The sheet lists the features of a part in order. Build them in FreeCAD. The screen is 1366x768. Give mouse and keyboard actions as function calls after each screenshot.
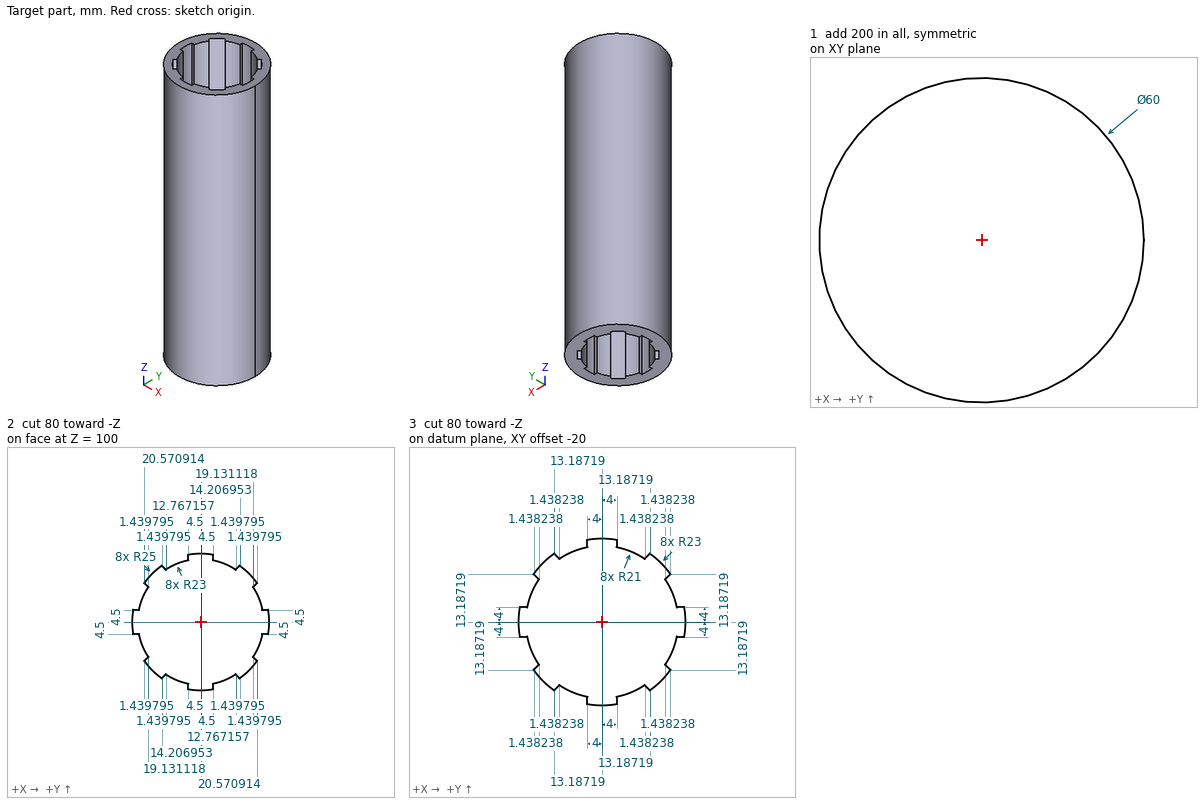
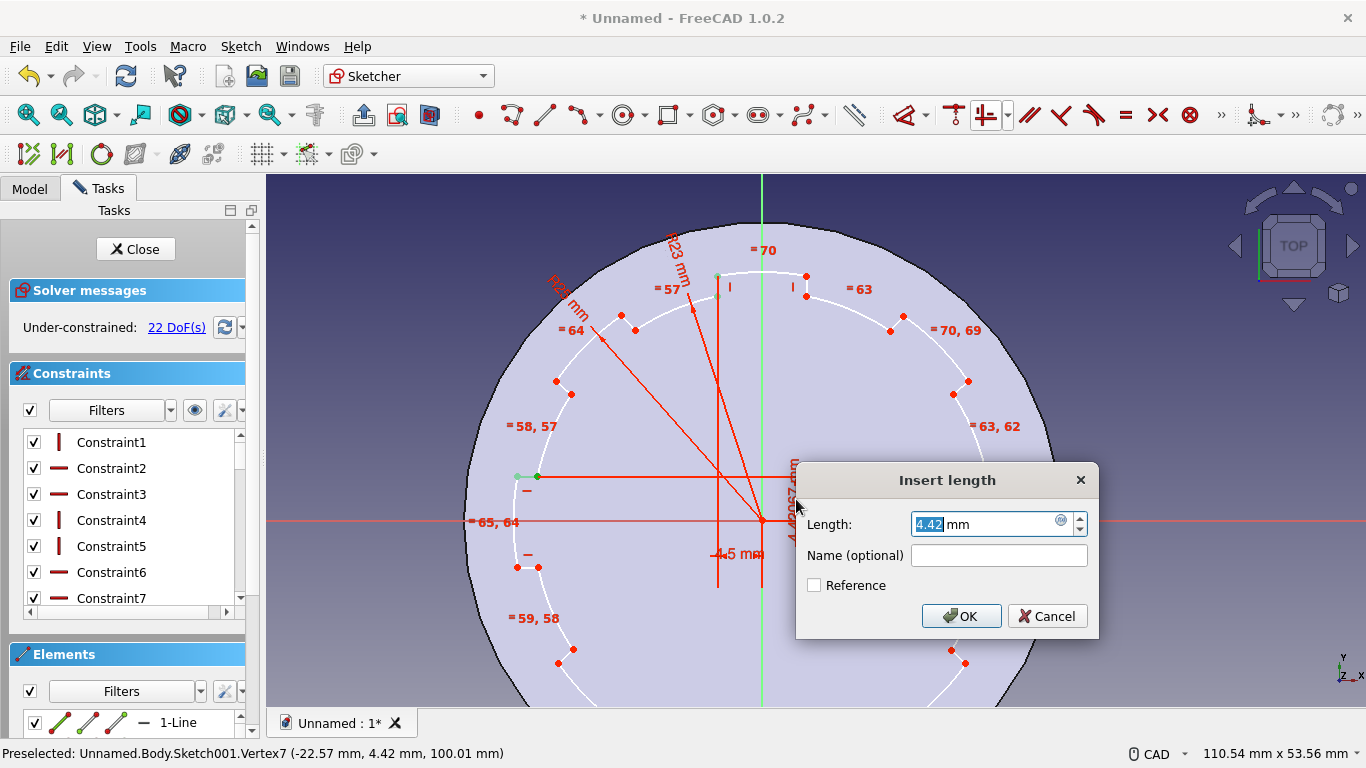
text(4.5)
key(Return)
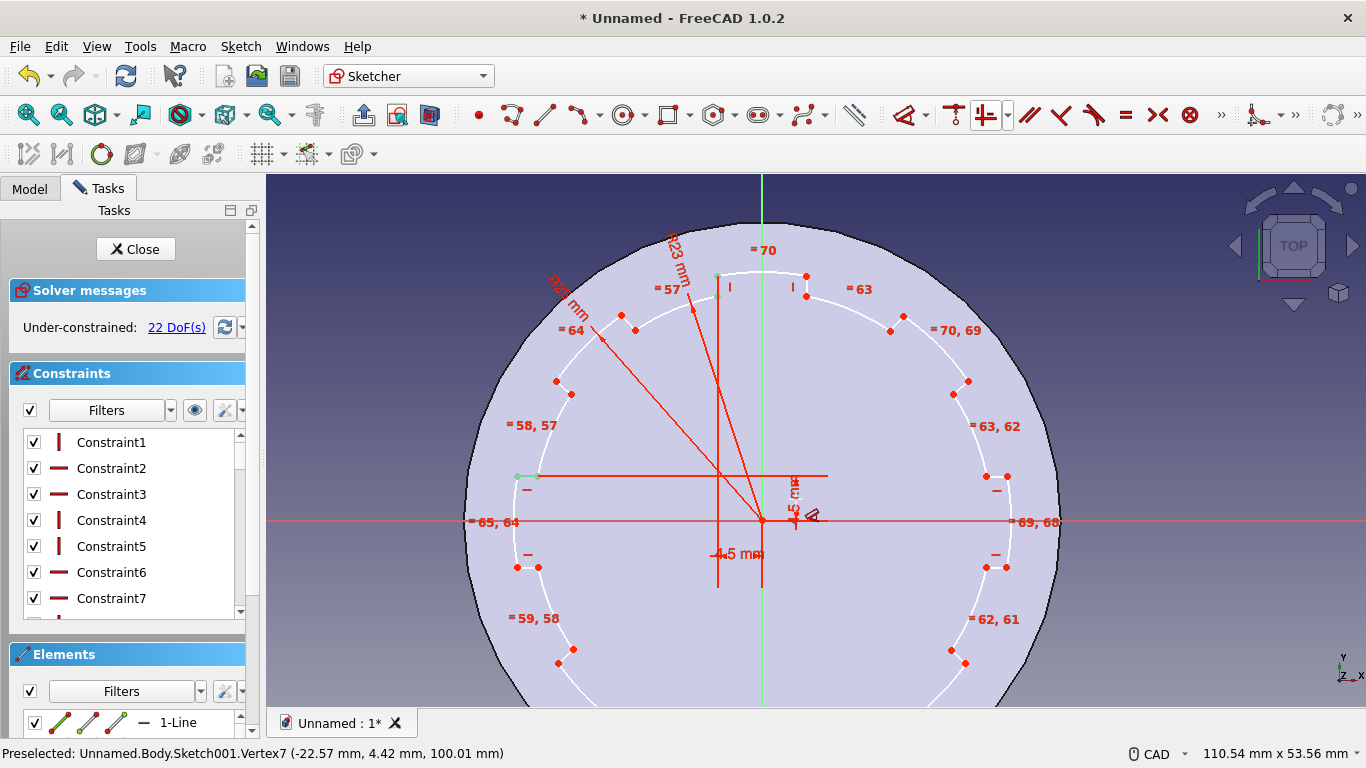
click(518, 568)
click(484, 544)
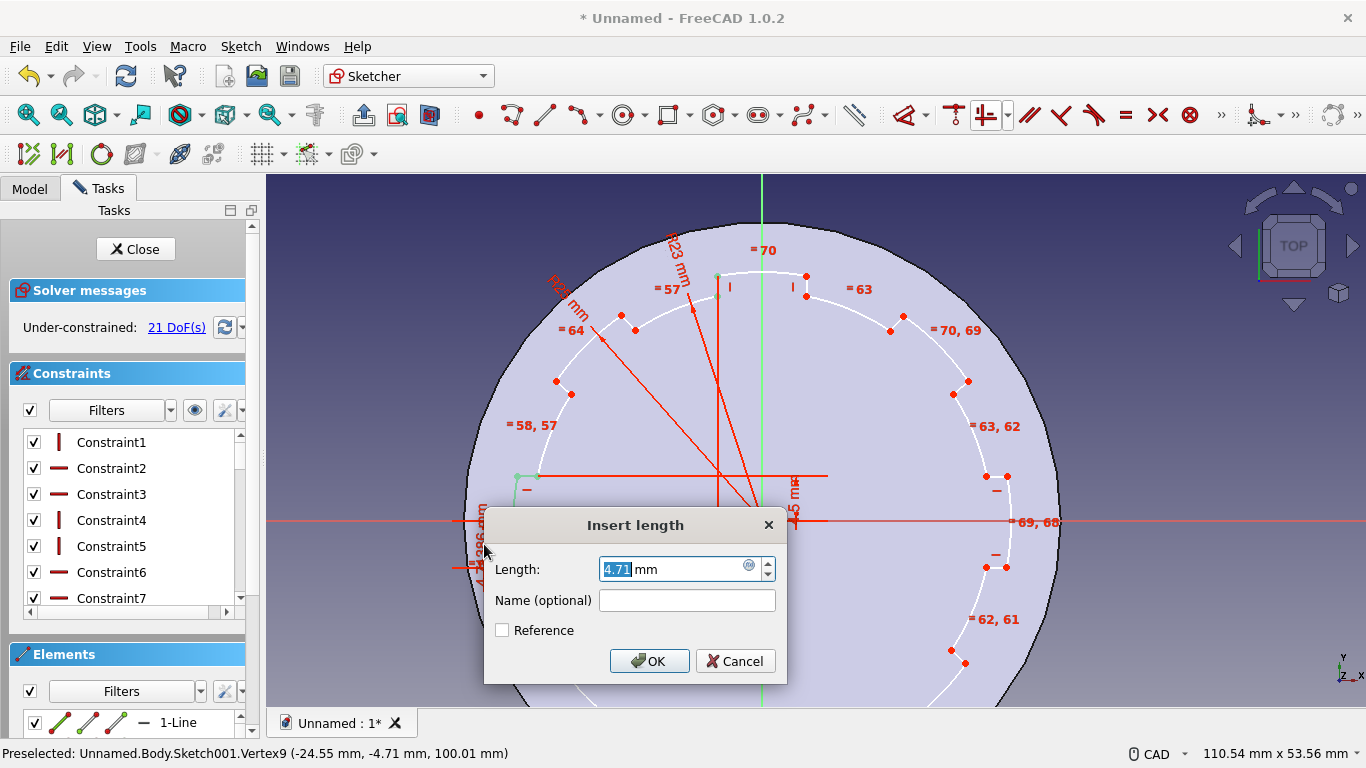
text(4.5)
key(Return)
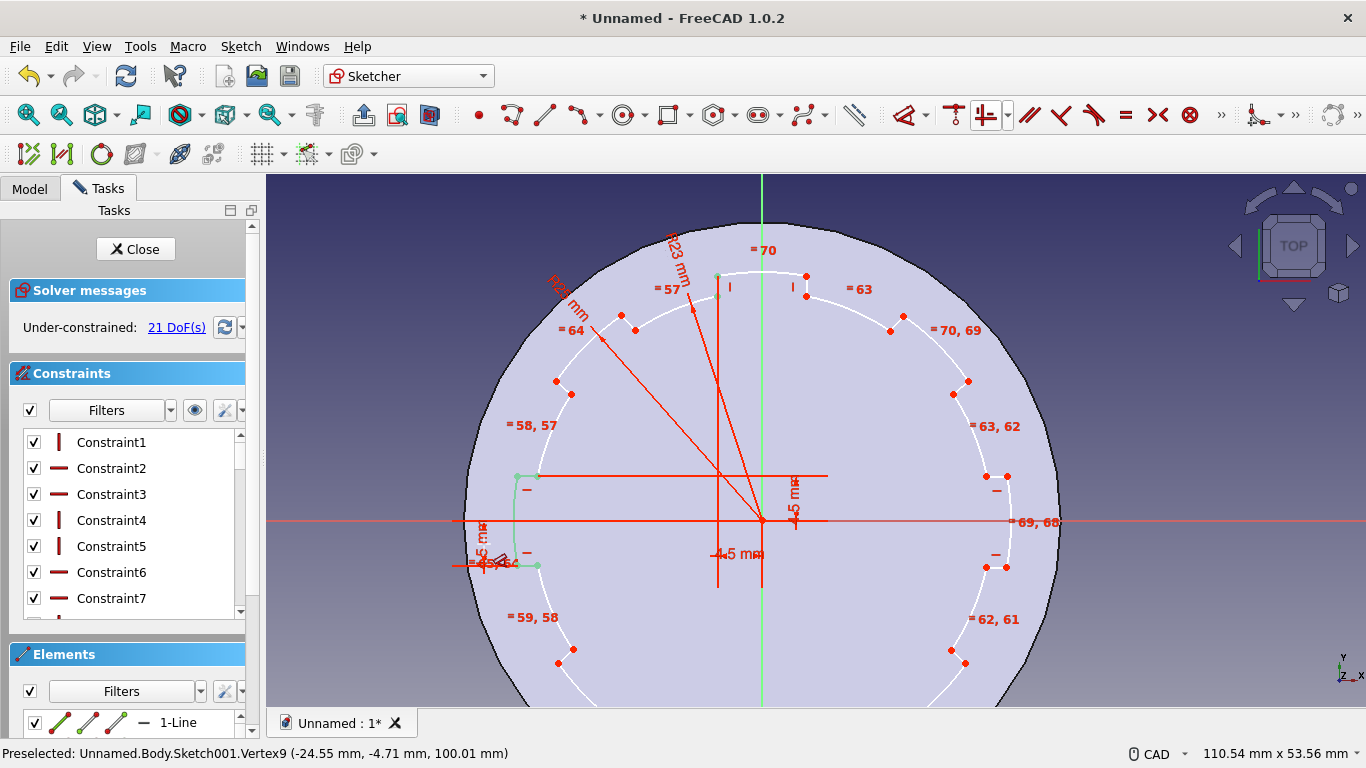
scroll(717, 277, down, 2)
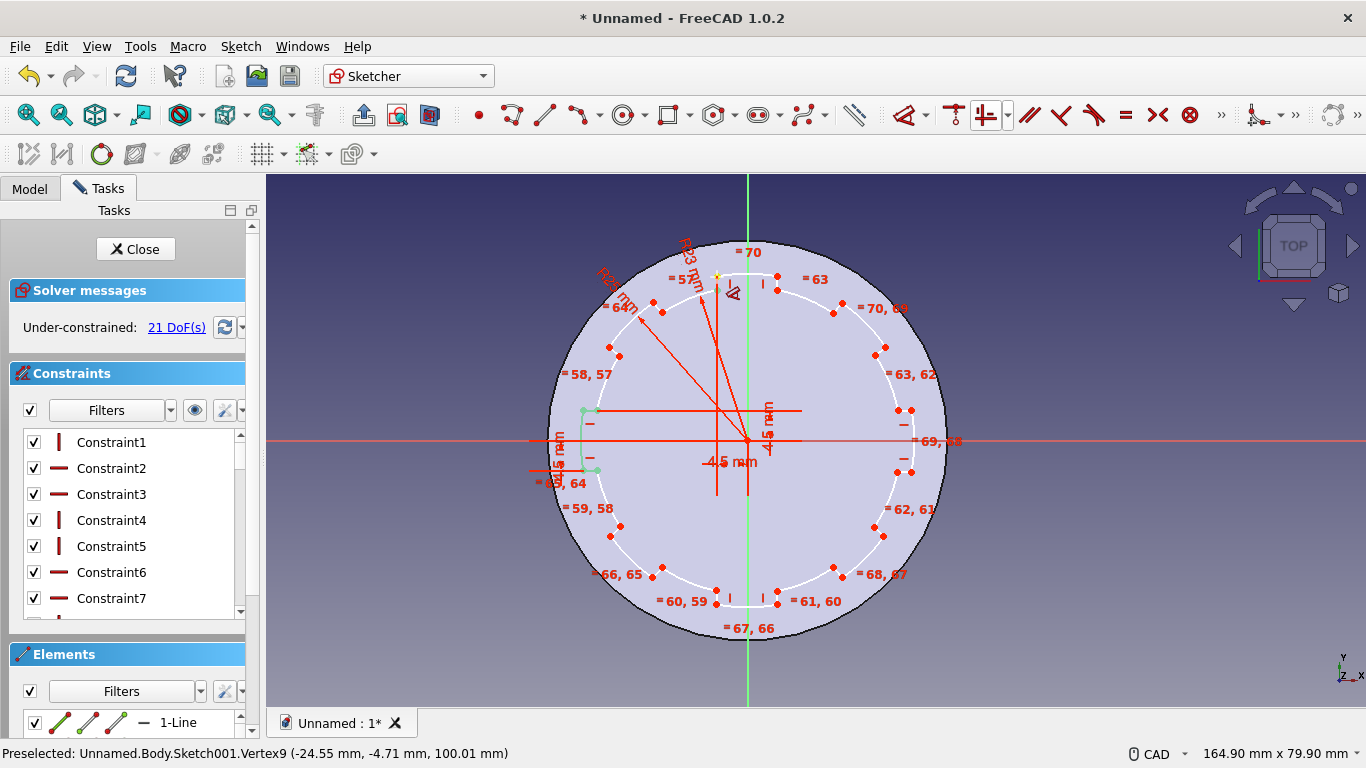
scroll(717, 591, up, 2)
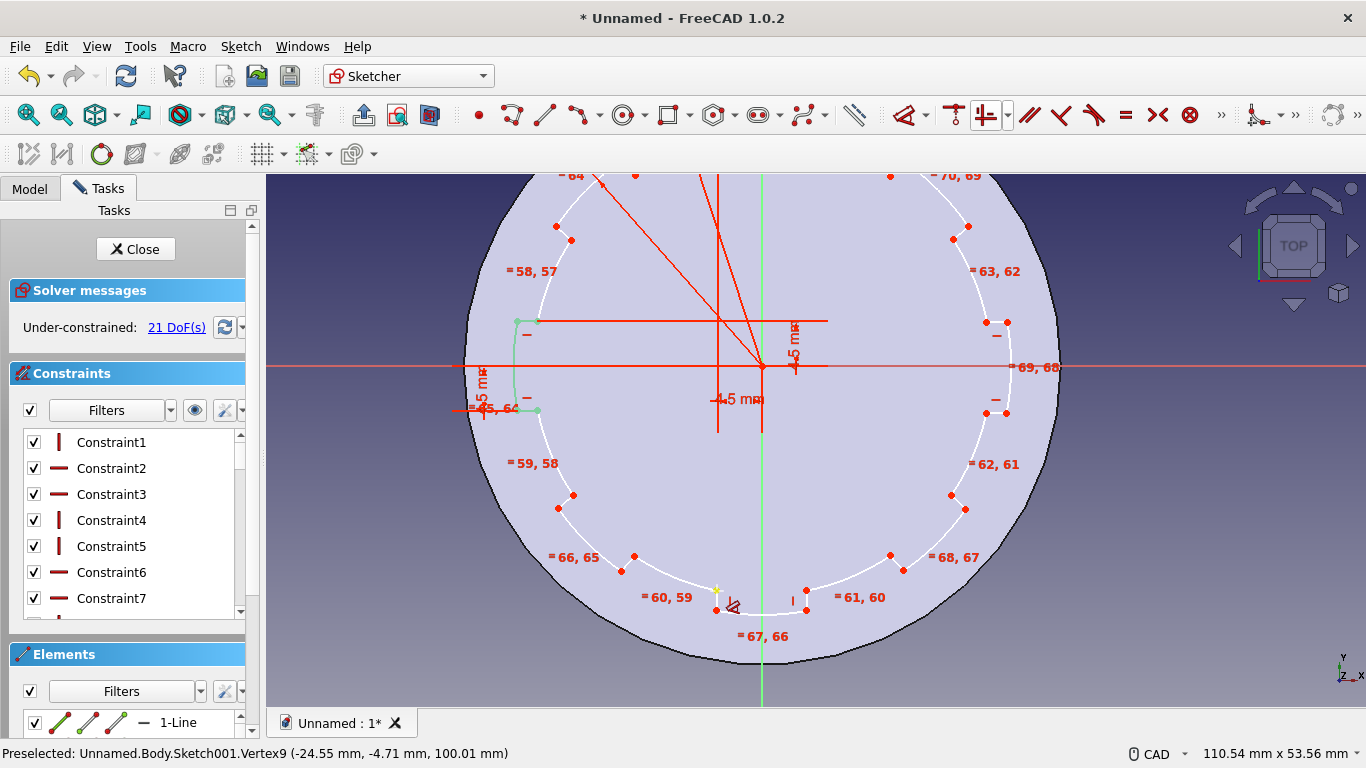
click(717, 590)
click(724, 332)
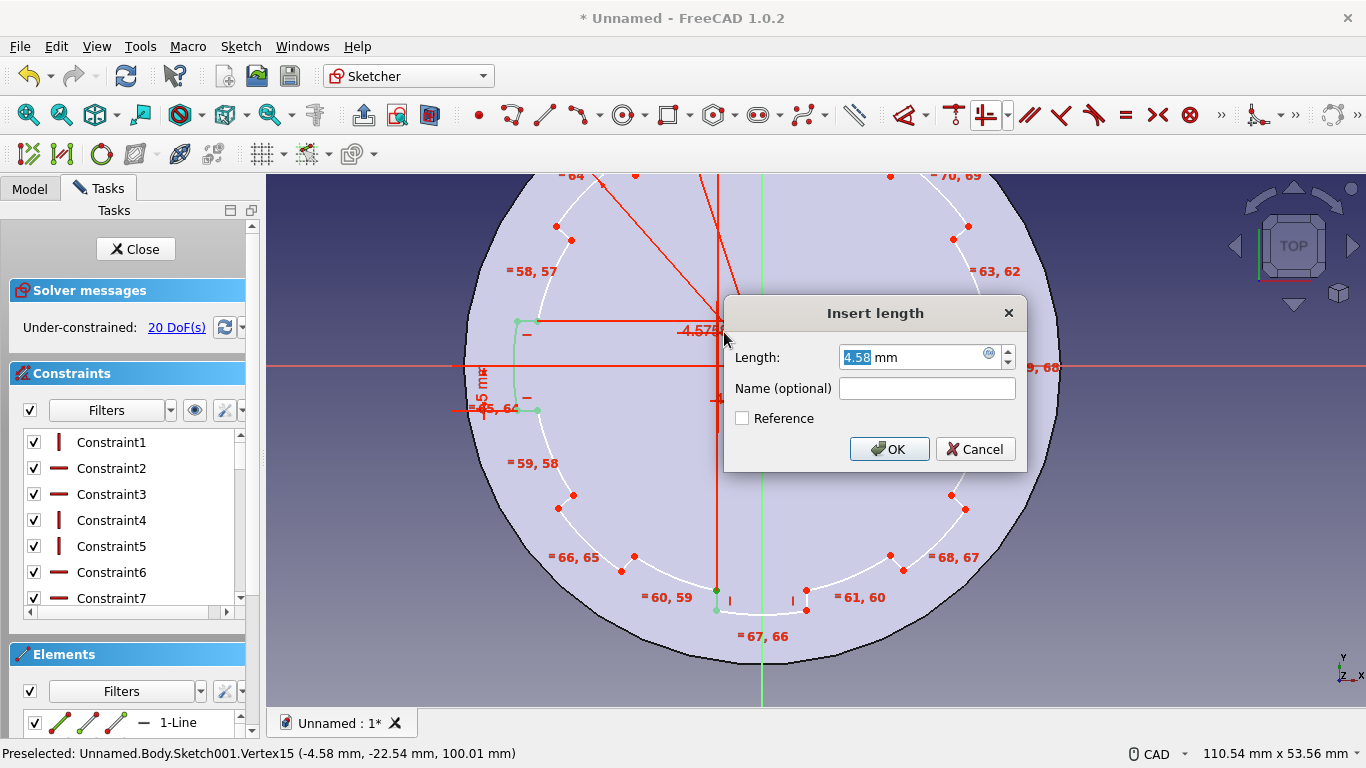
text(4.5)
key(Return)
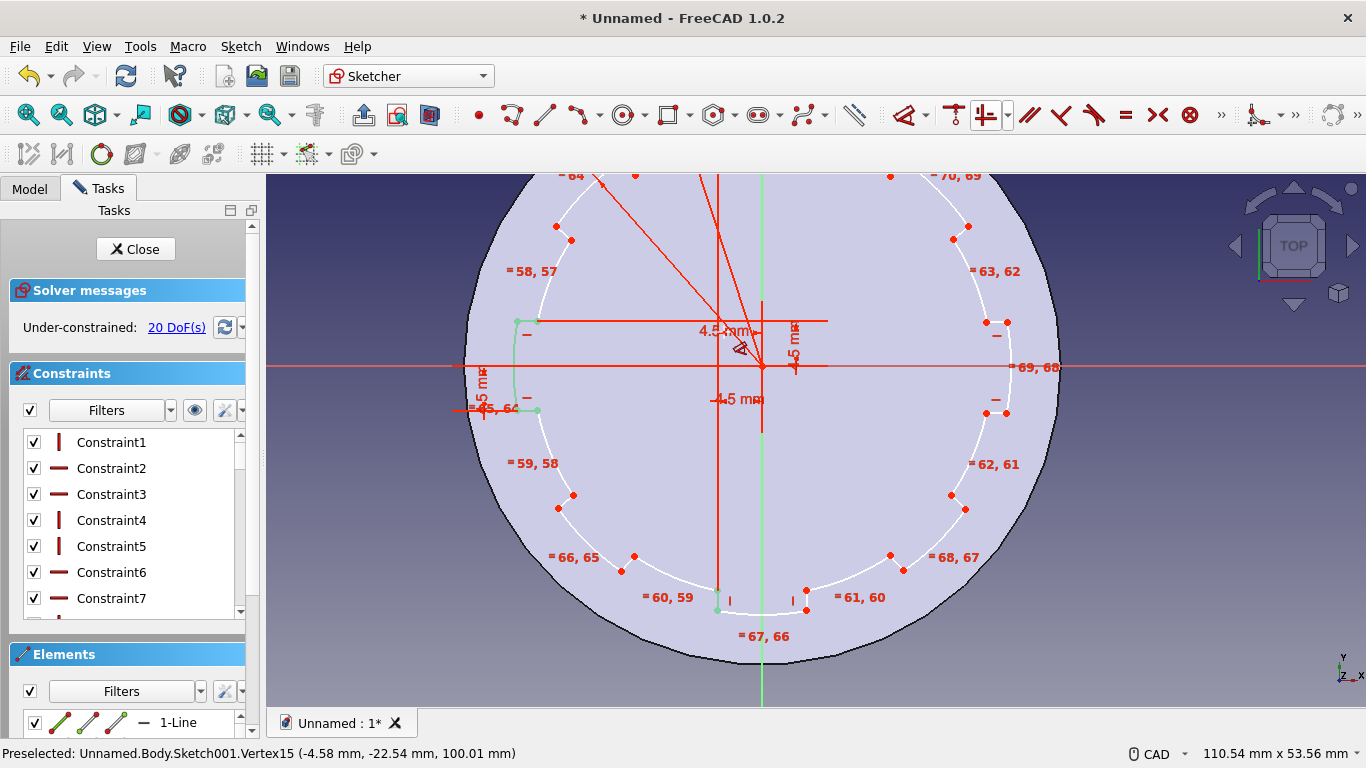
click(807, 611)
click(784, 645)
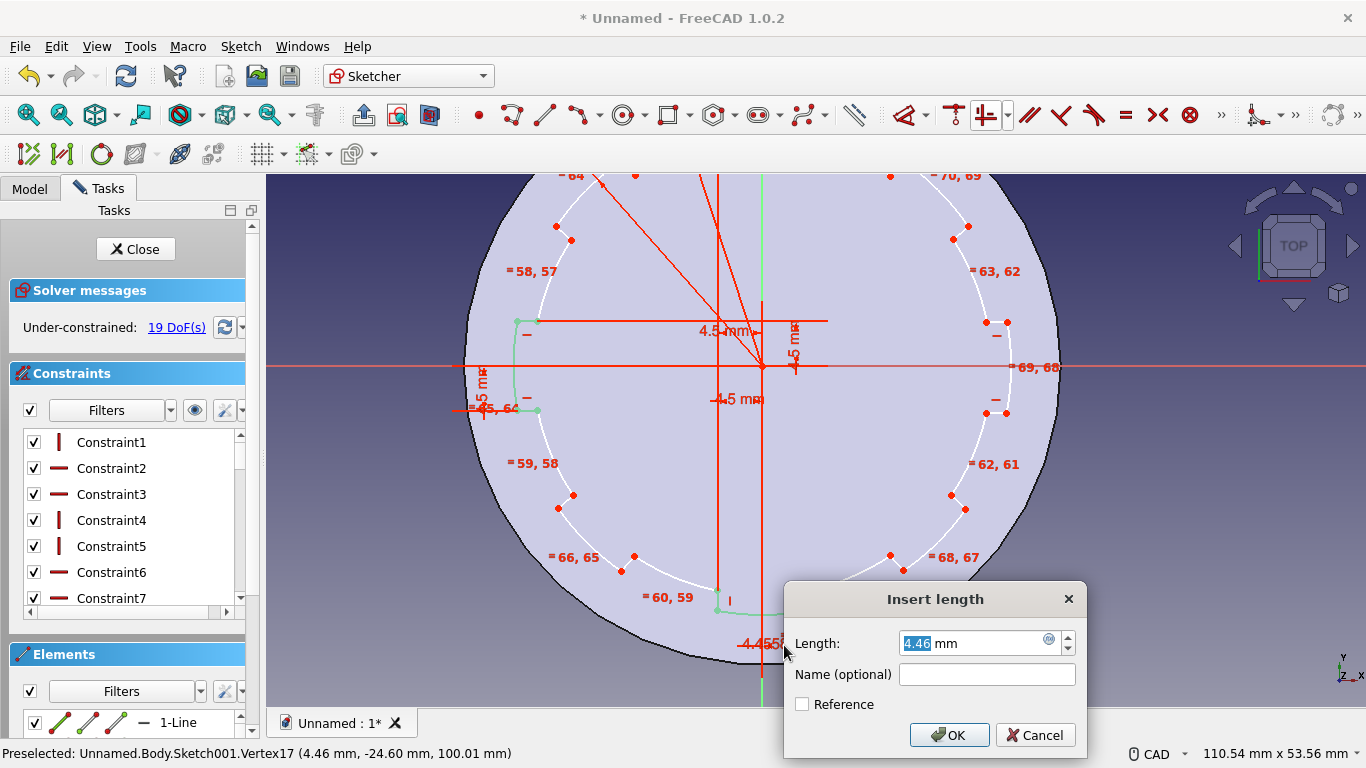
text(4.5)
key(Return)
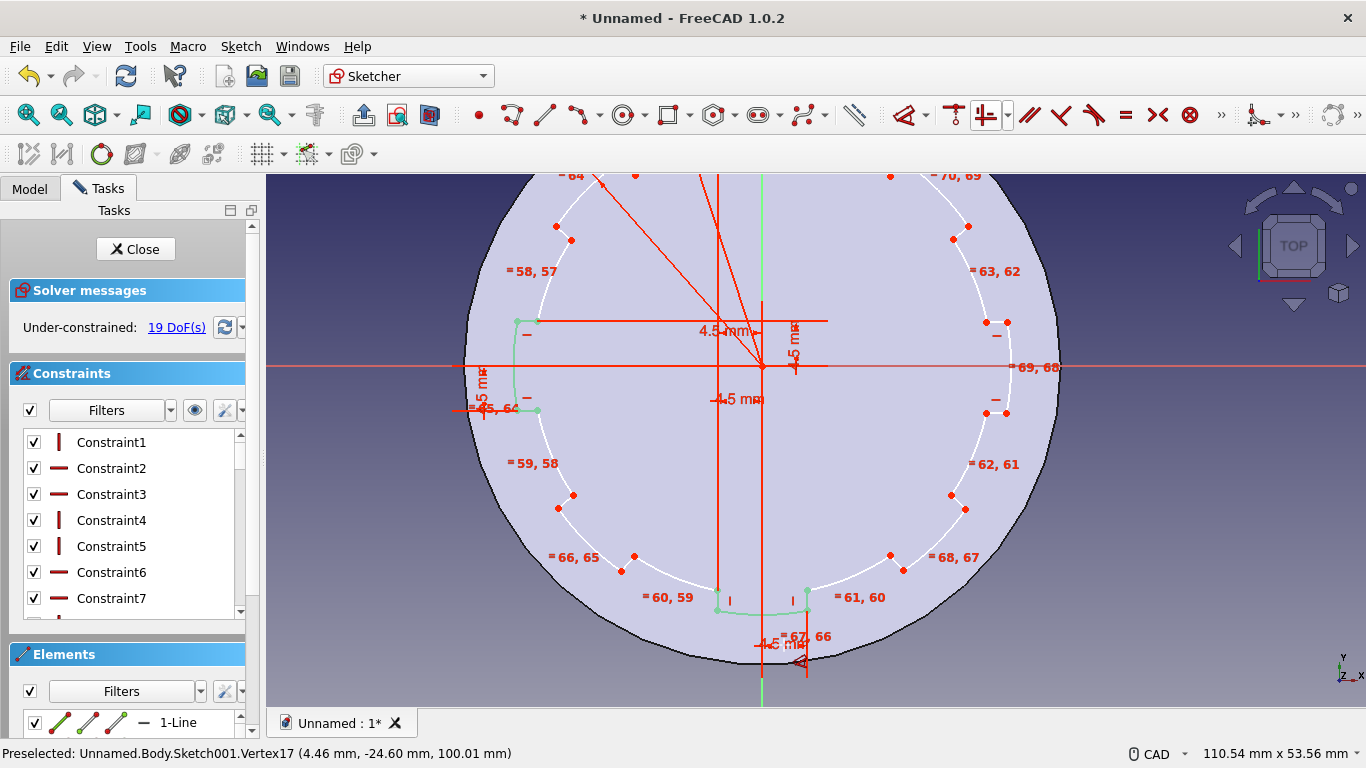
click(986, 413)
click(1044, 390)